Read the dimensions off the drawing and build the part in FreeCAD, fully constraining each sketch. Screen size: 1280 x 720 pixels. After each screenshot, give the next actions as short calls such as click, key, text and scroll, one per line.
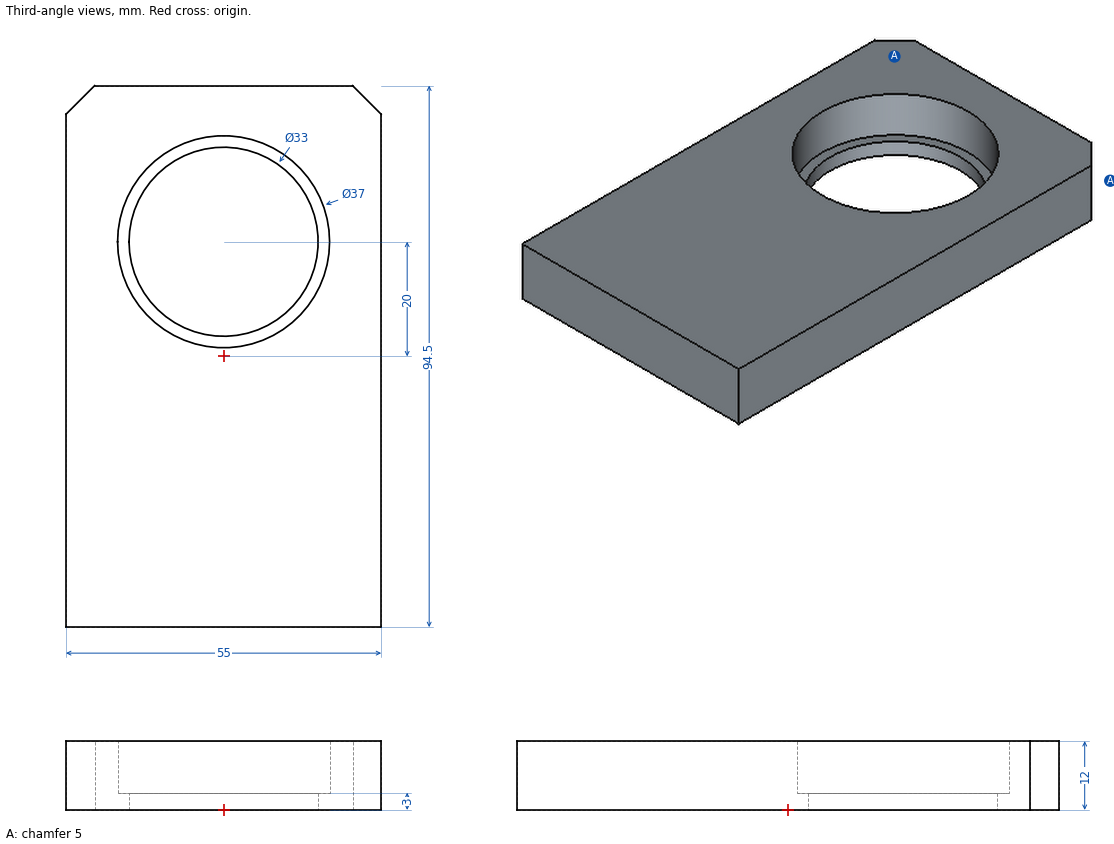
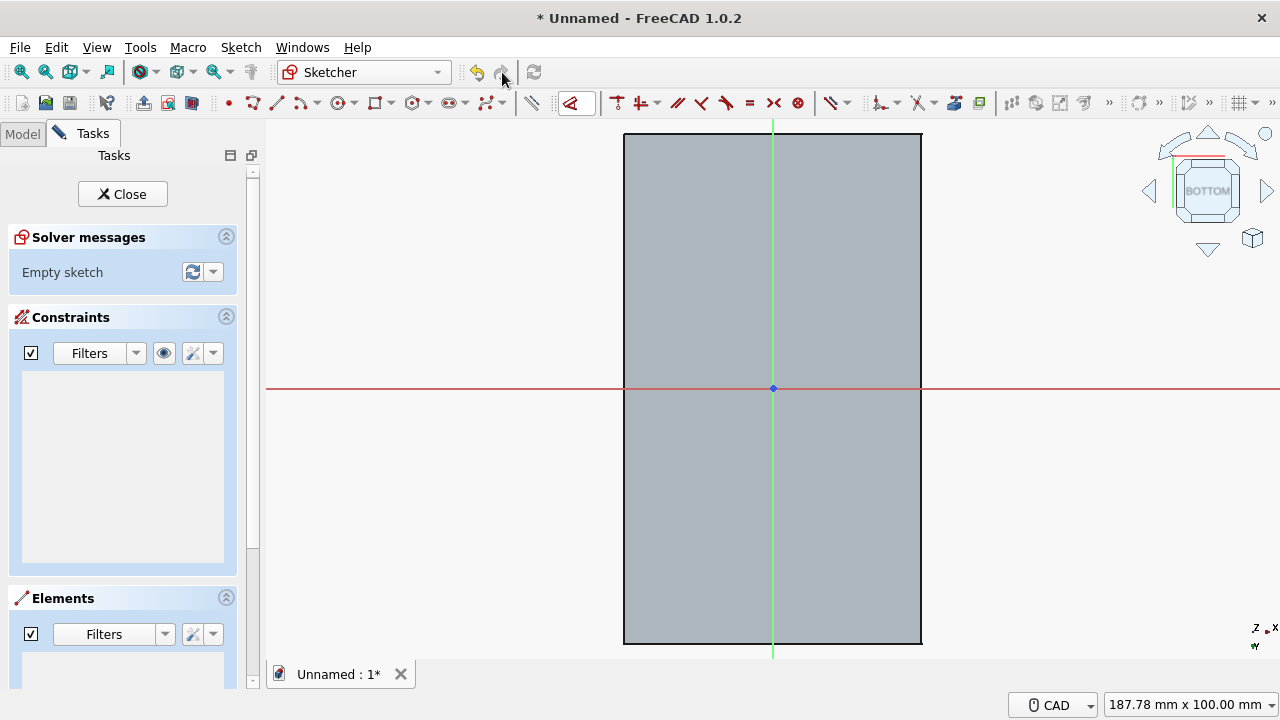
scroll(912, 631, up, 2)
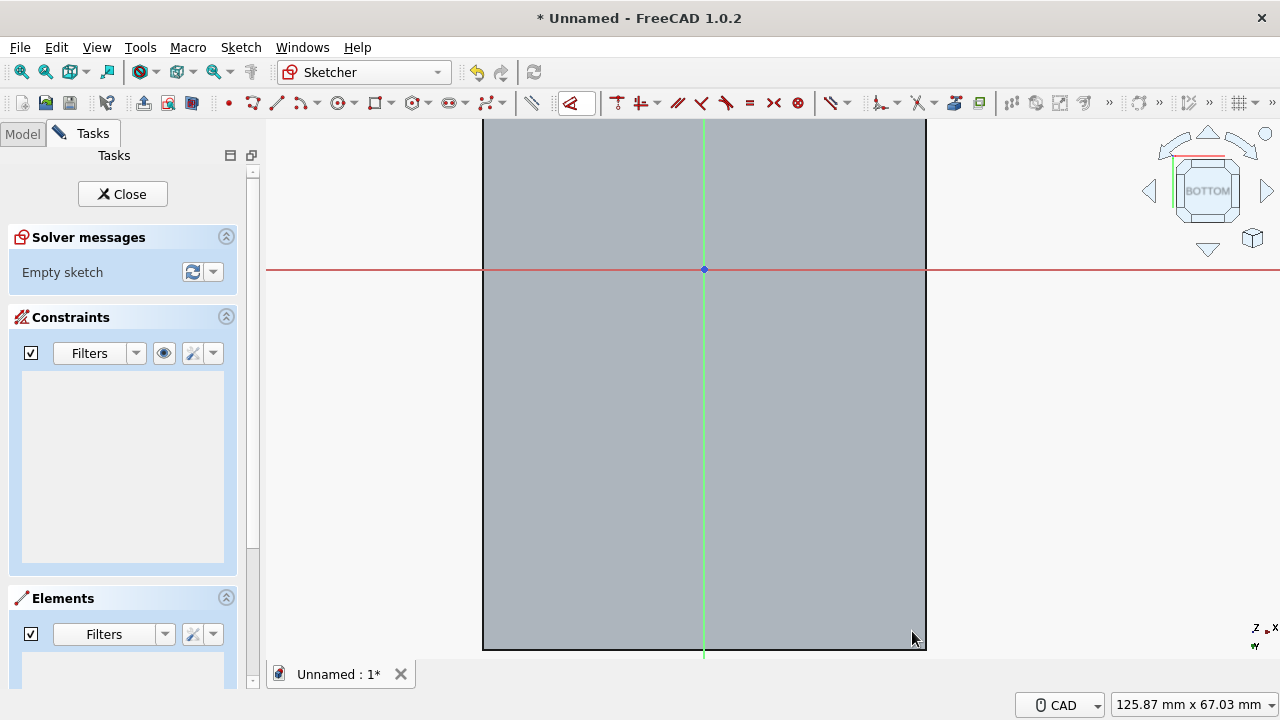
click(338, 104)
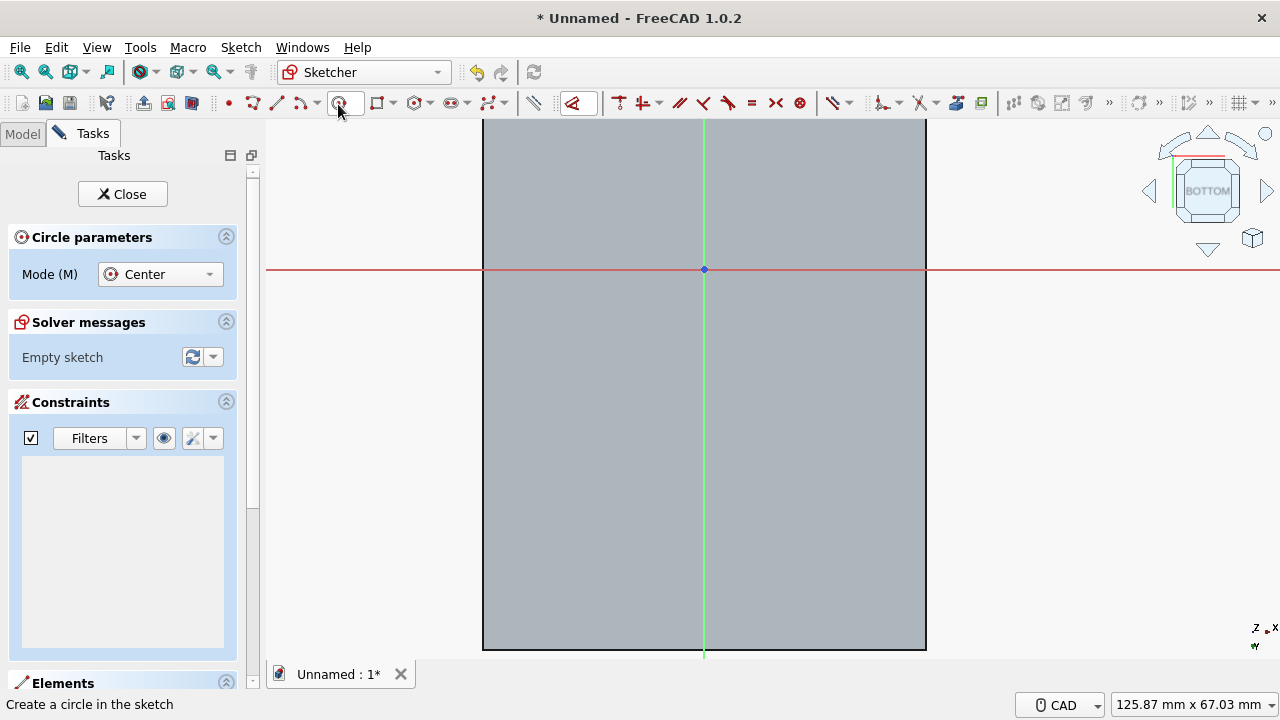
click(704, 431)
click(810, 325)
key(Escape)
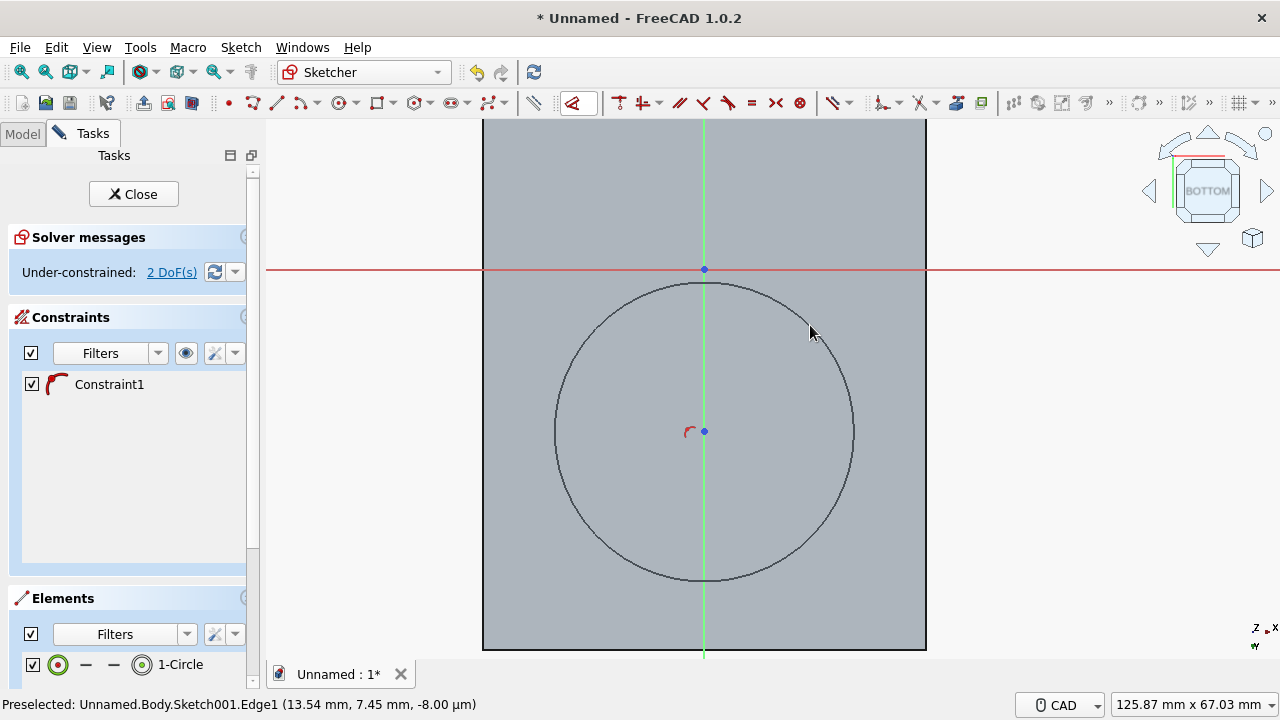
click(810, 326)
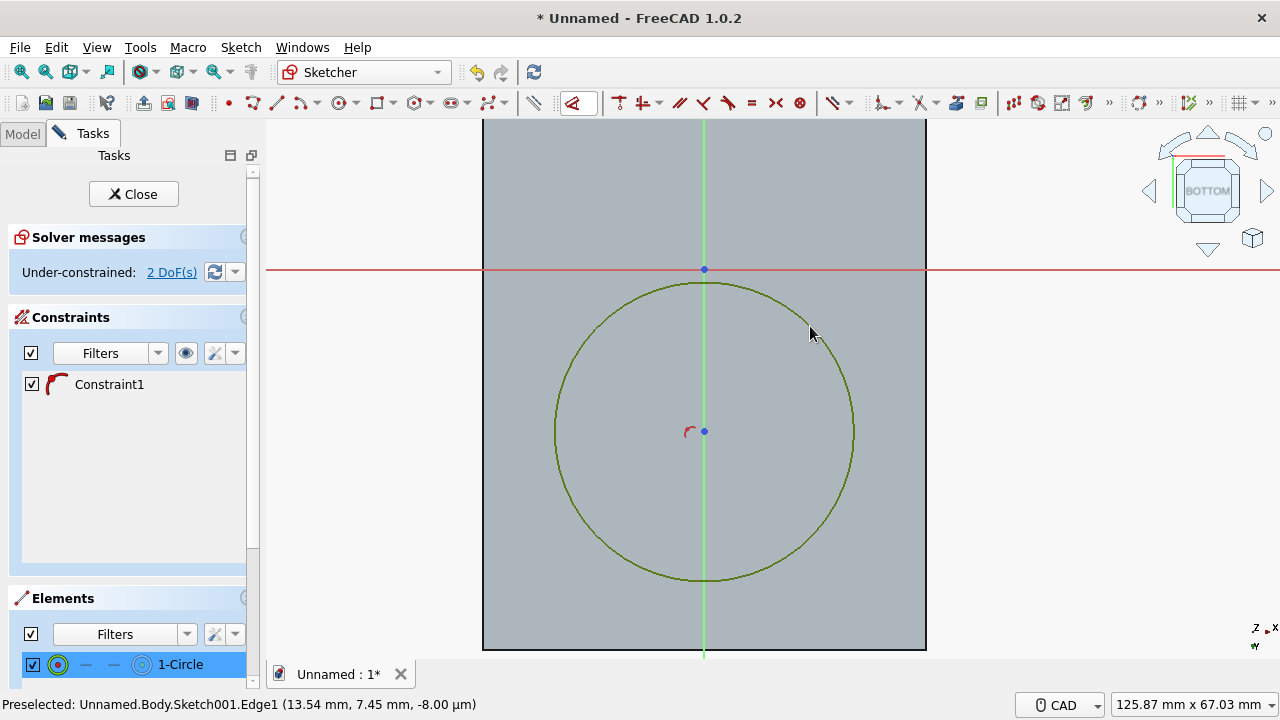
key(k)
key(o)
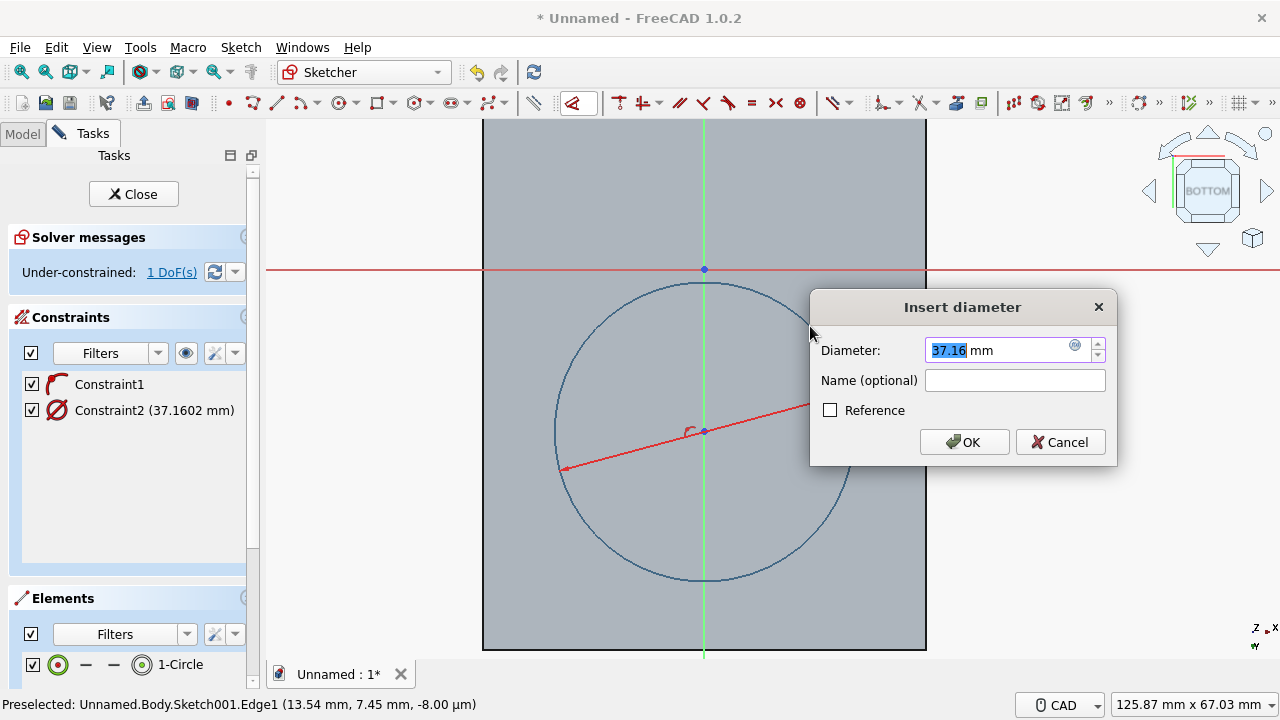
text(37)
key(Return)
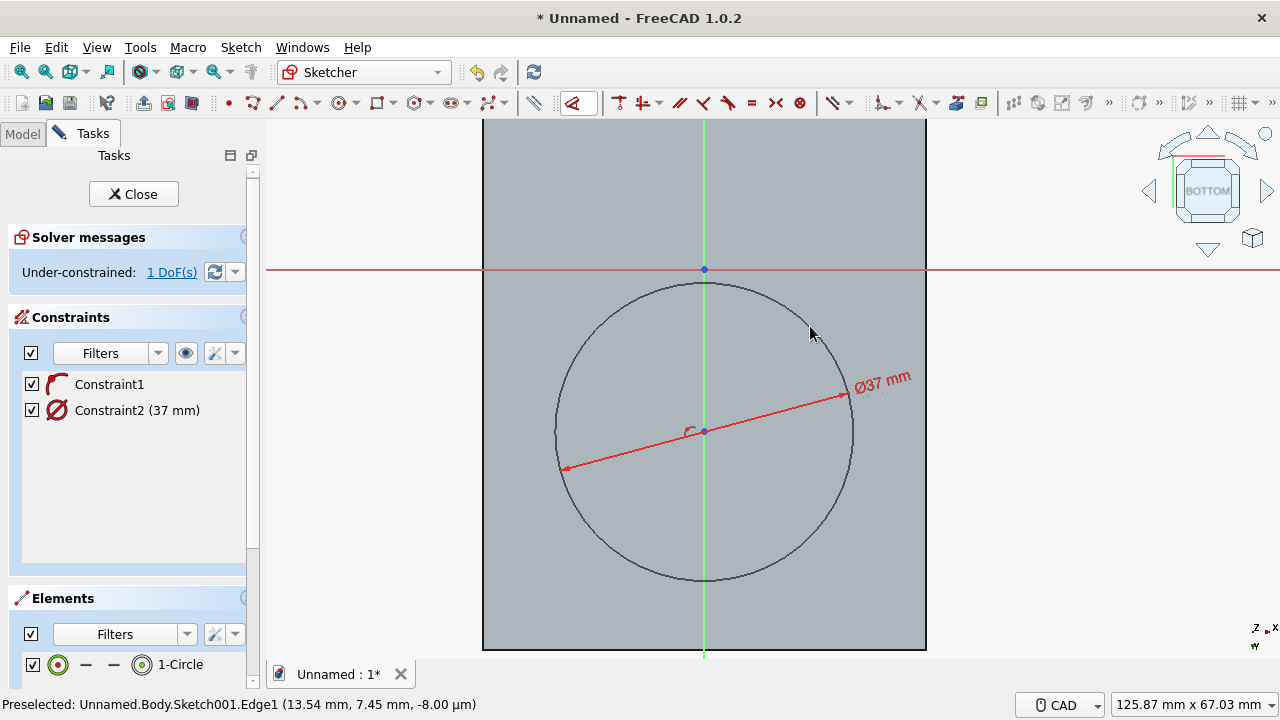
click(704, 432)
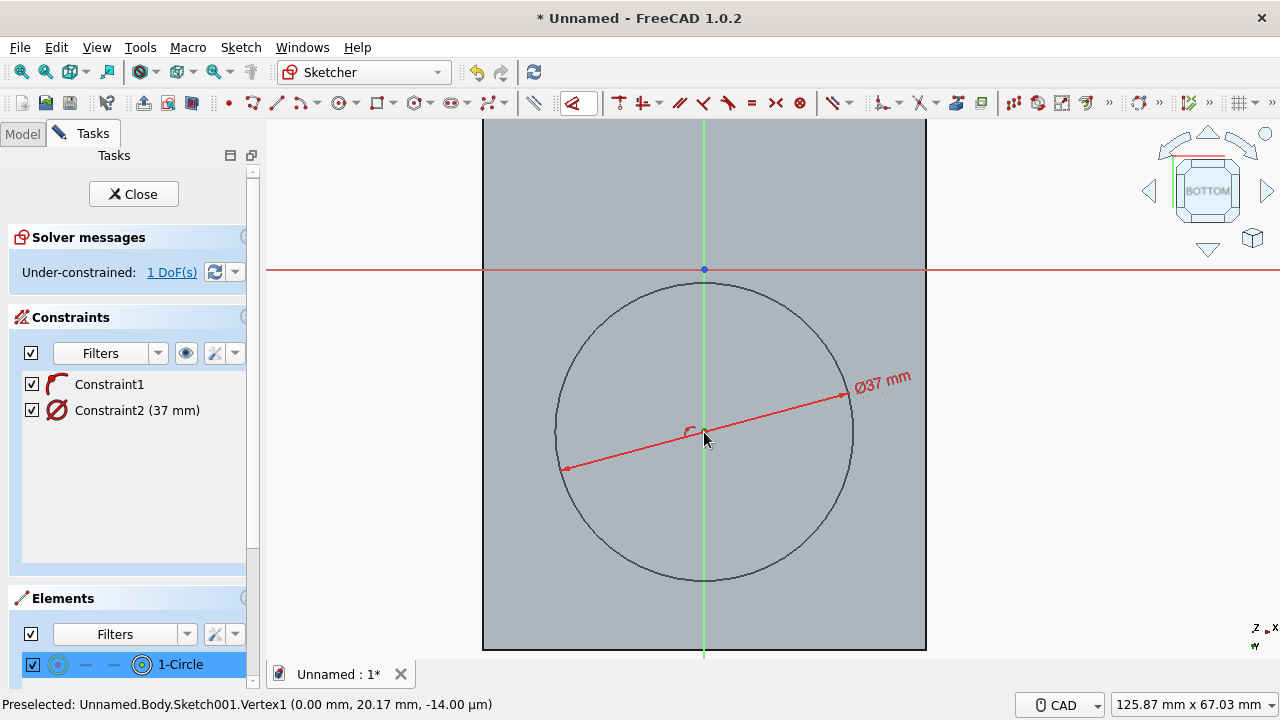
key(i)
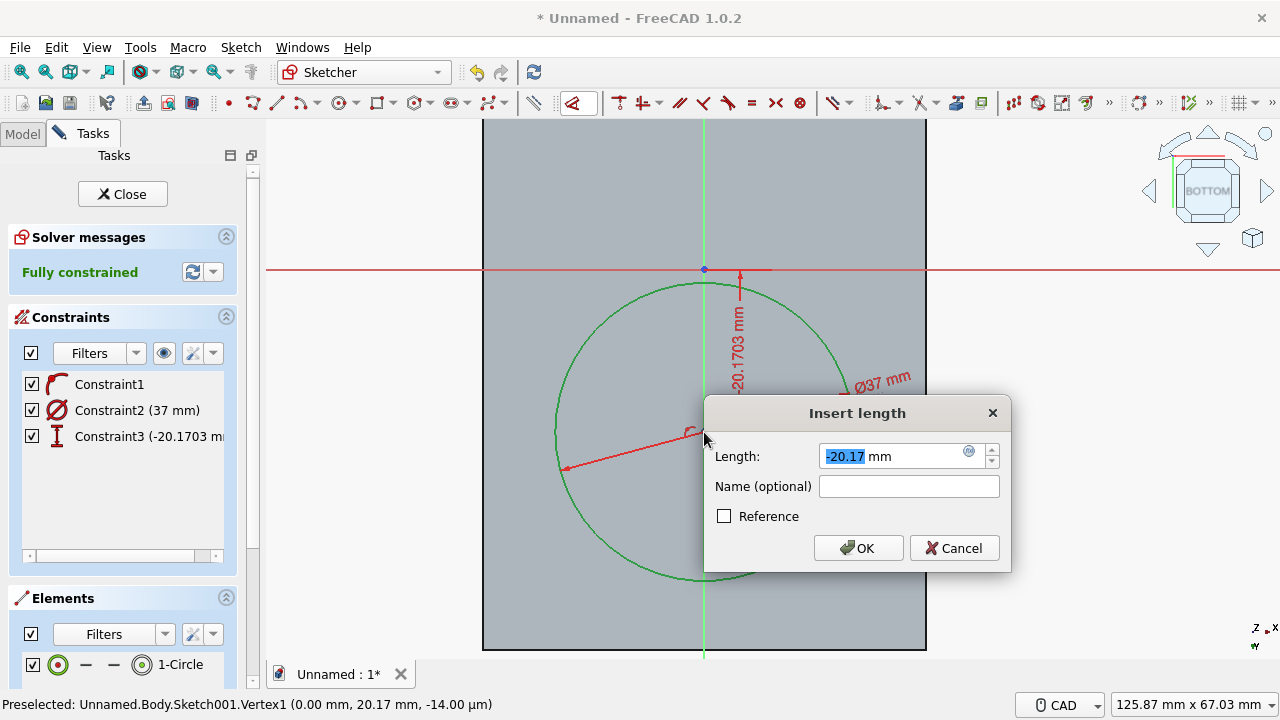
text(-20)
key(Return)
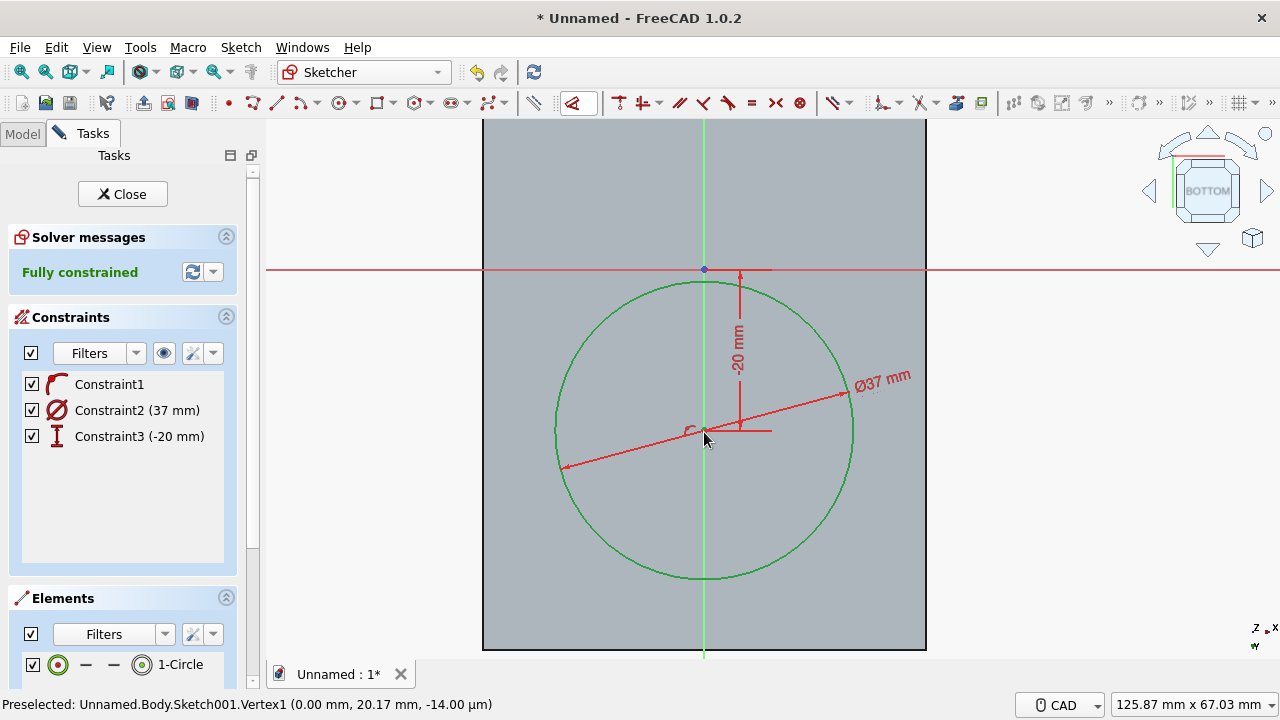
click(123, 194)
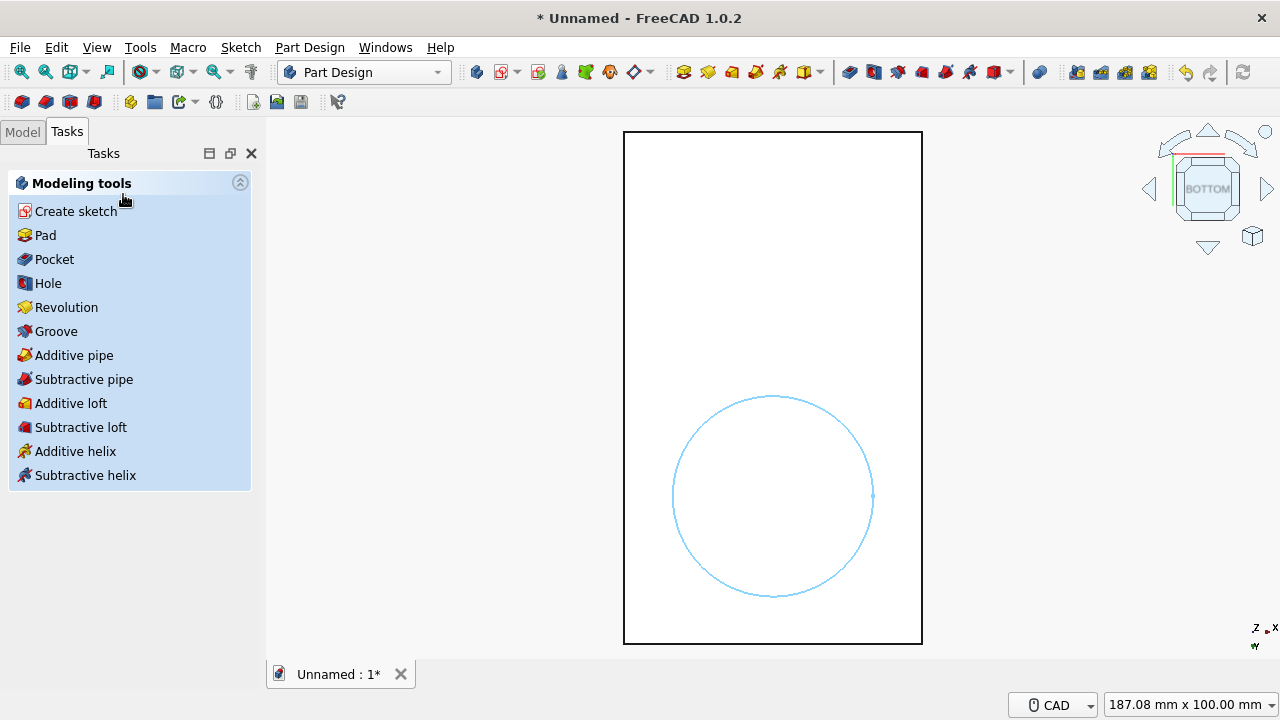
click(850, 72)